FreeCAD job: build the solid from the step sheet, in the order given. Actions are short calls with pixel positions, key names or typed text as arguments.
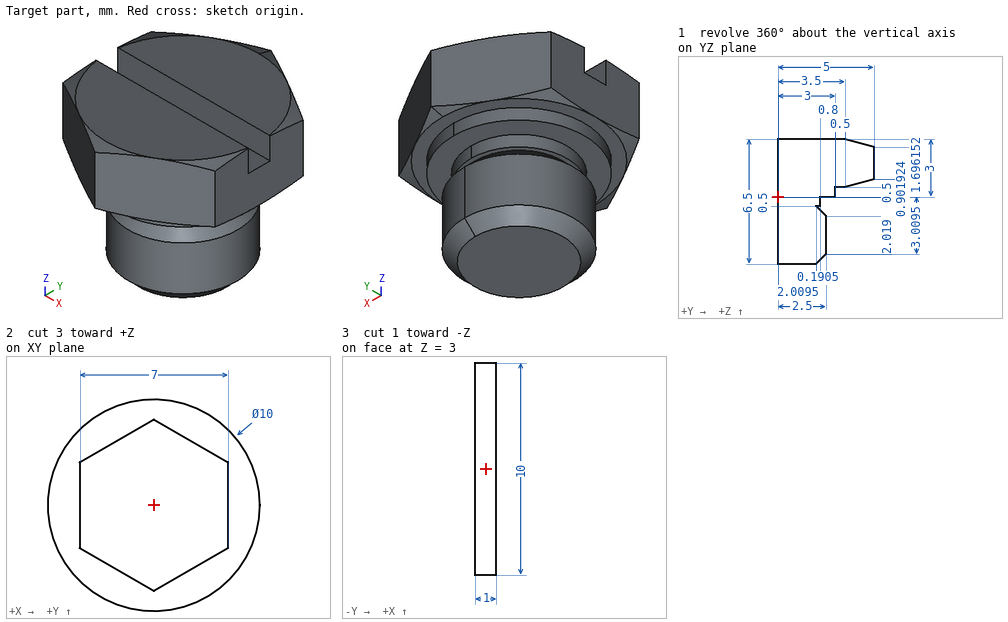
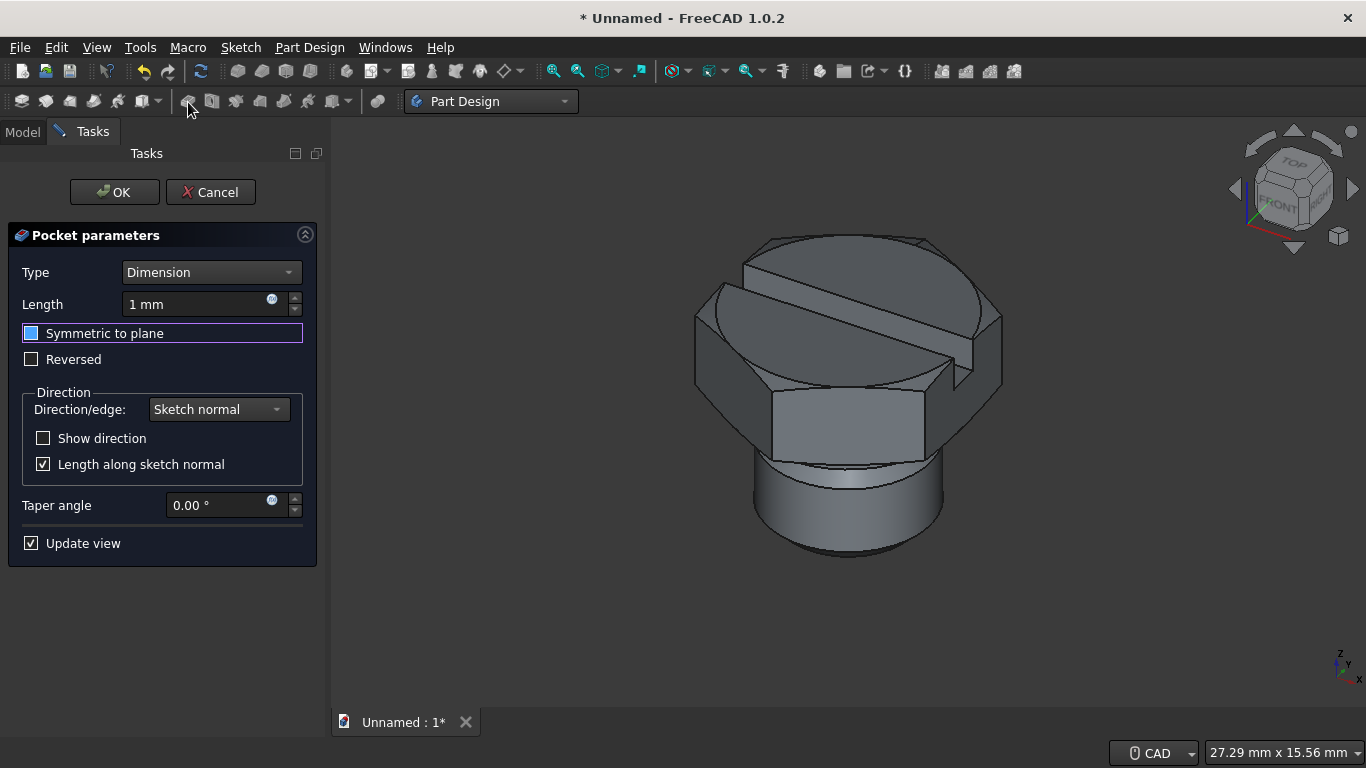
click(115, 192)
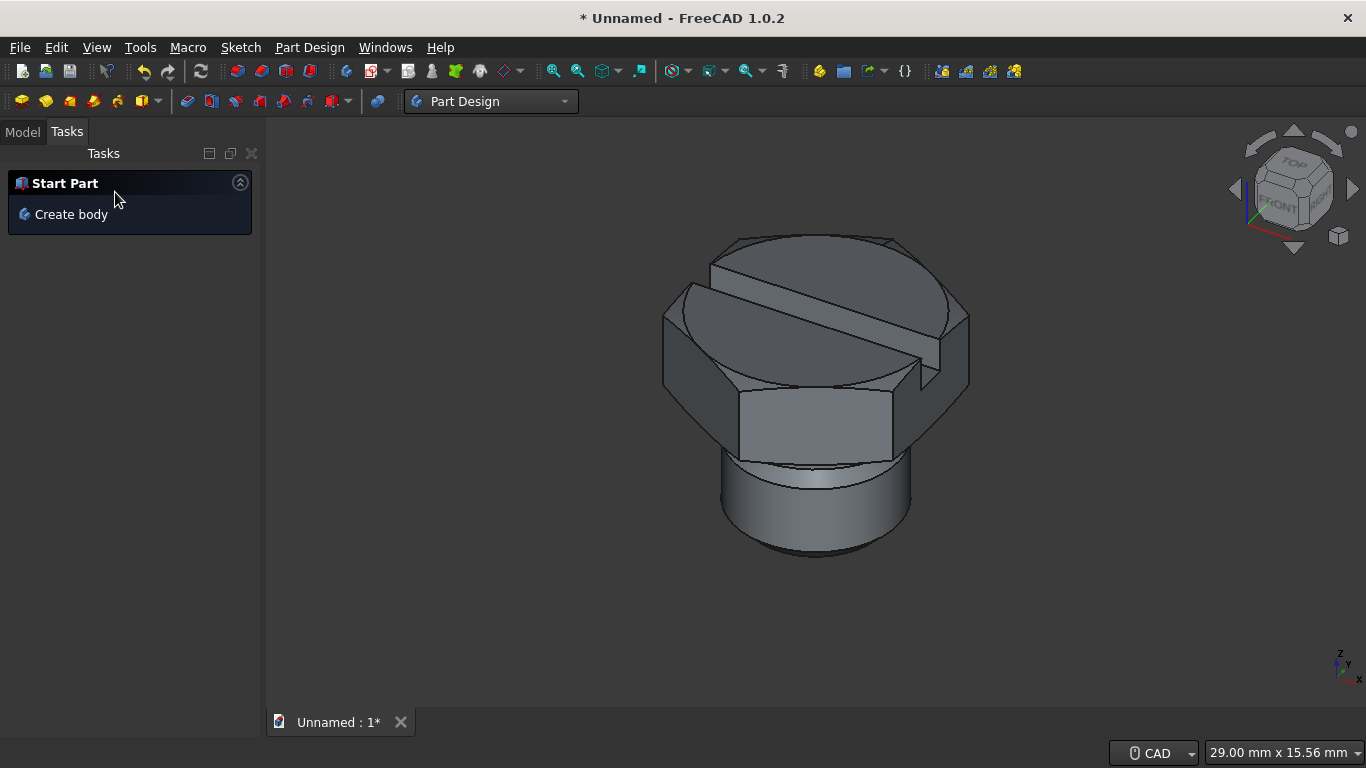
key(0)